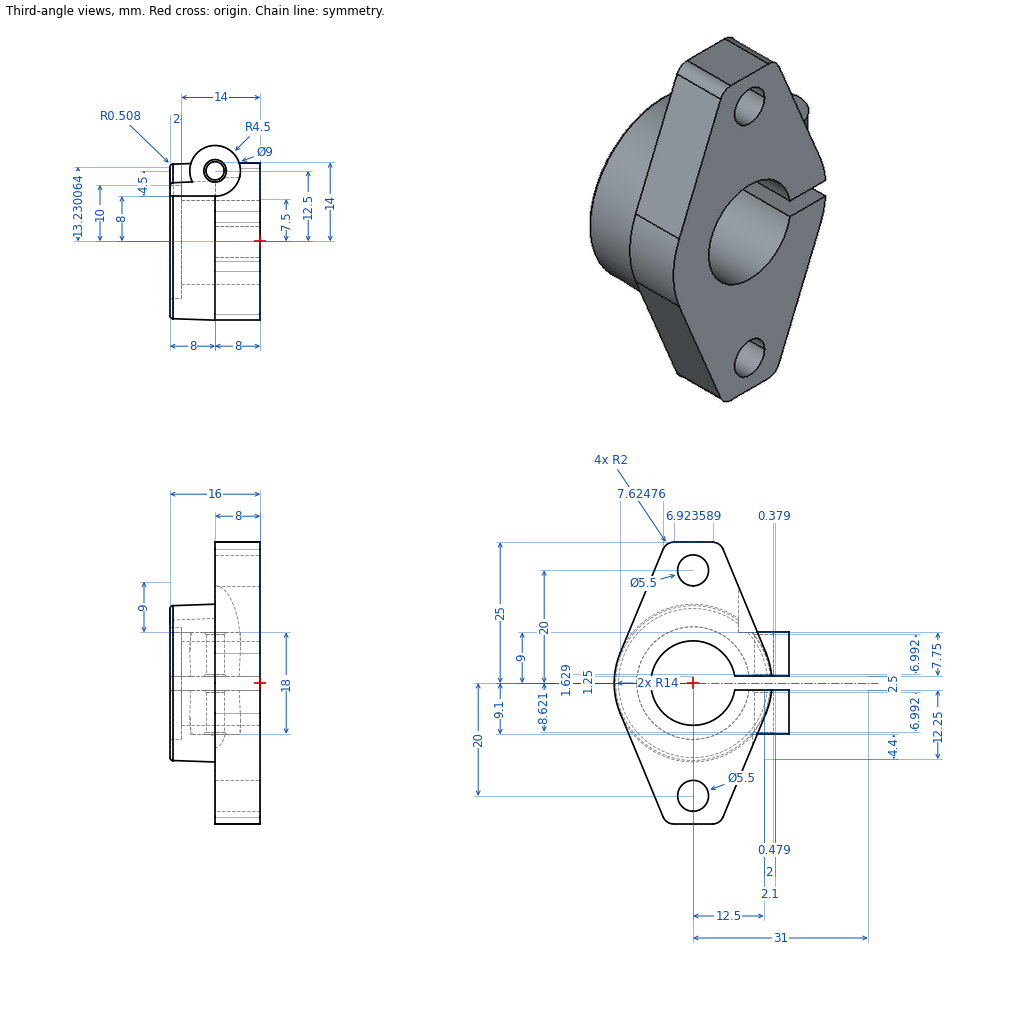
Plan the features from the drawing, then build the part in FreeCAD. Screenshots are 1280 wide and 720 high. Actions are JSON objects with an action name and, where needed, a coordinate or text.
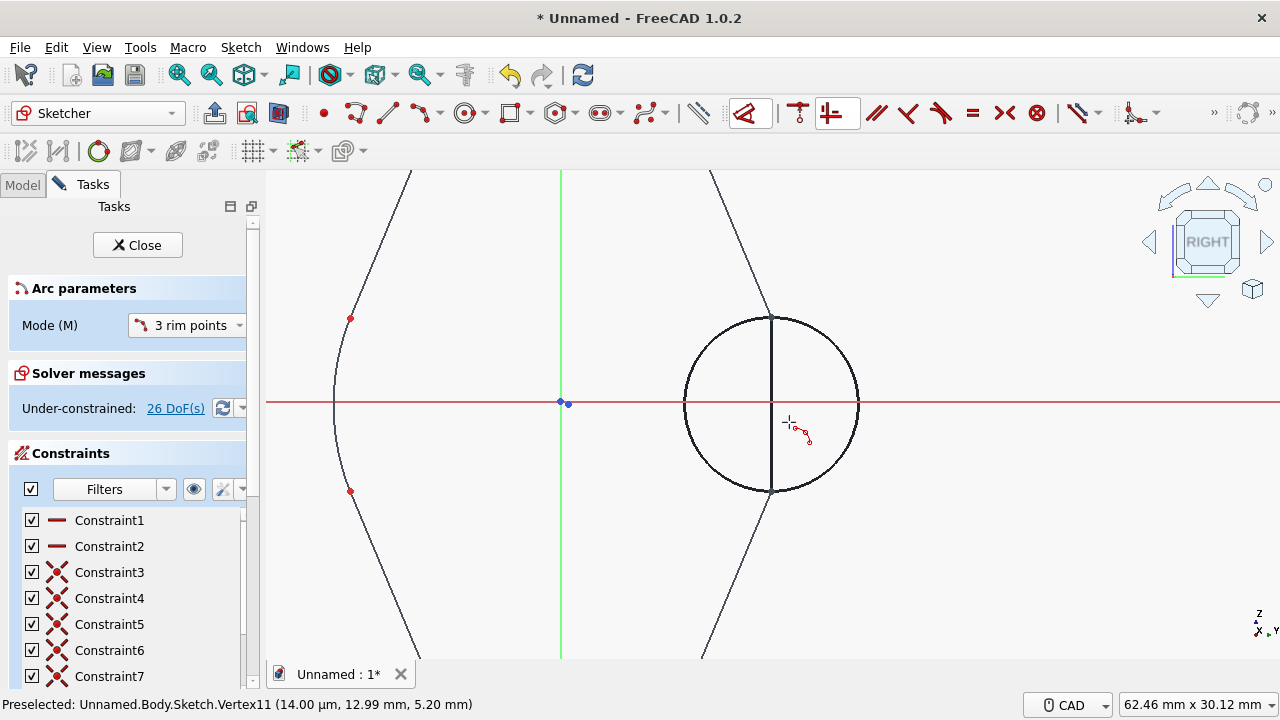
{"action": "left_click", "coordinate": [787, 420]}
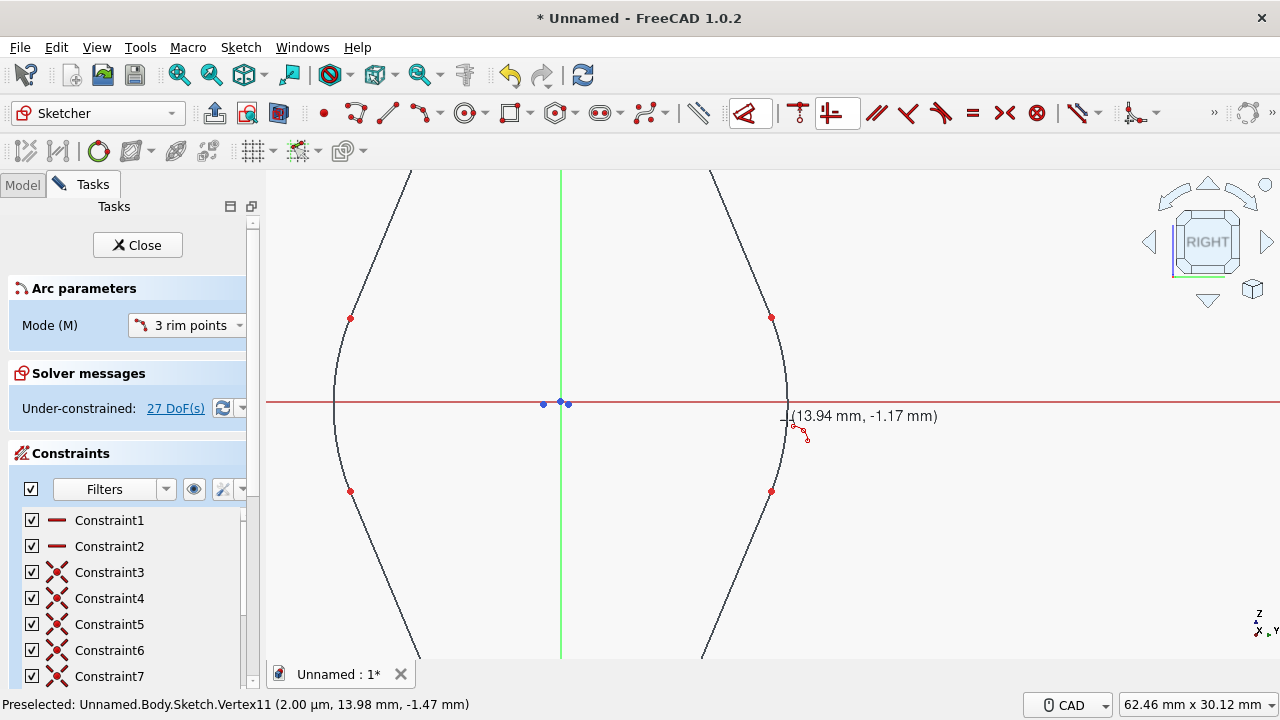
{"action": "scroll", "coordinate": [788, 422], "scroll_direction": "down", "scroll_amount": 5}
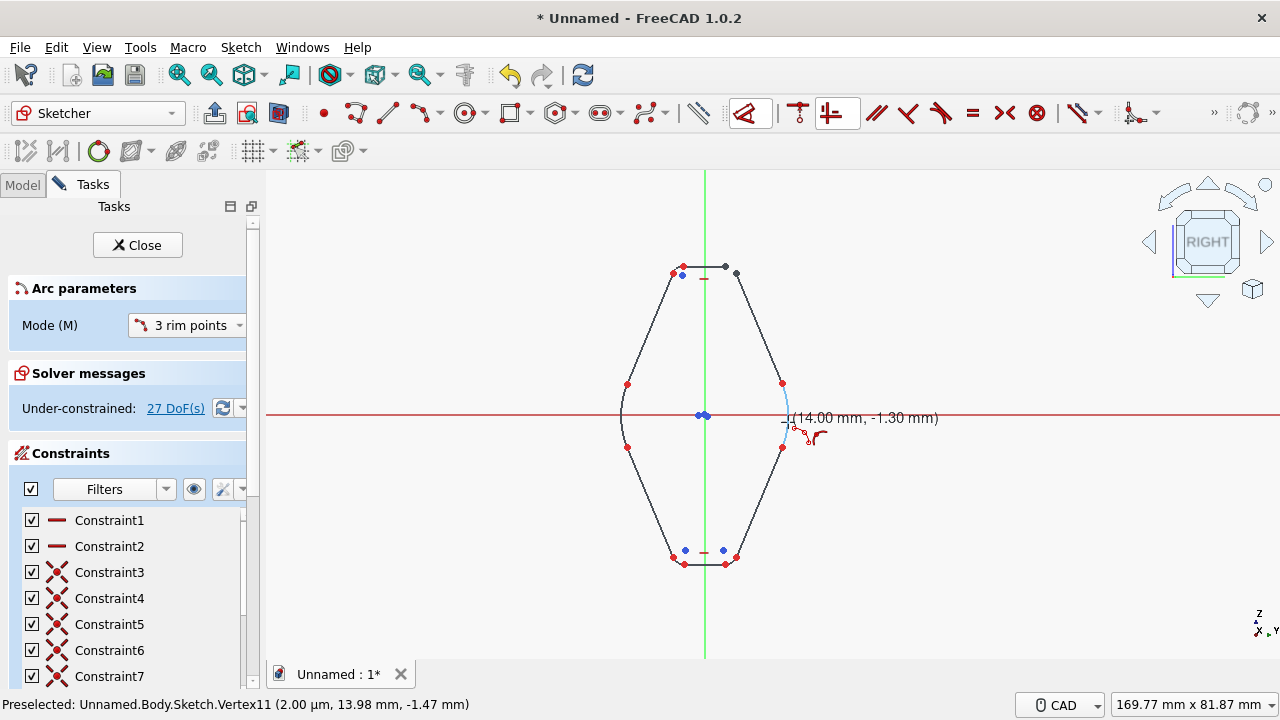
{"action": "left_click", "coordinate": [736, 274]}
{"action": "left_click", "coordinate": [725, 267]}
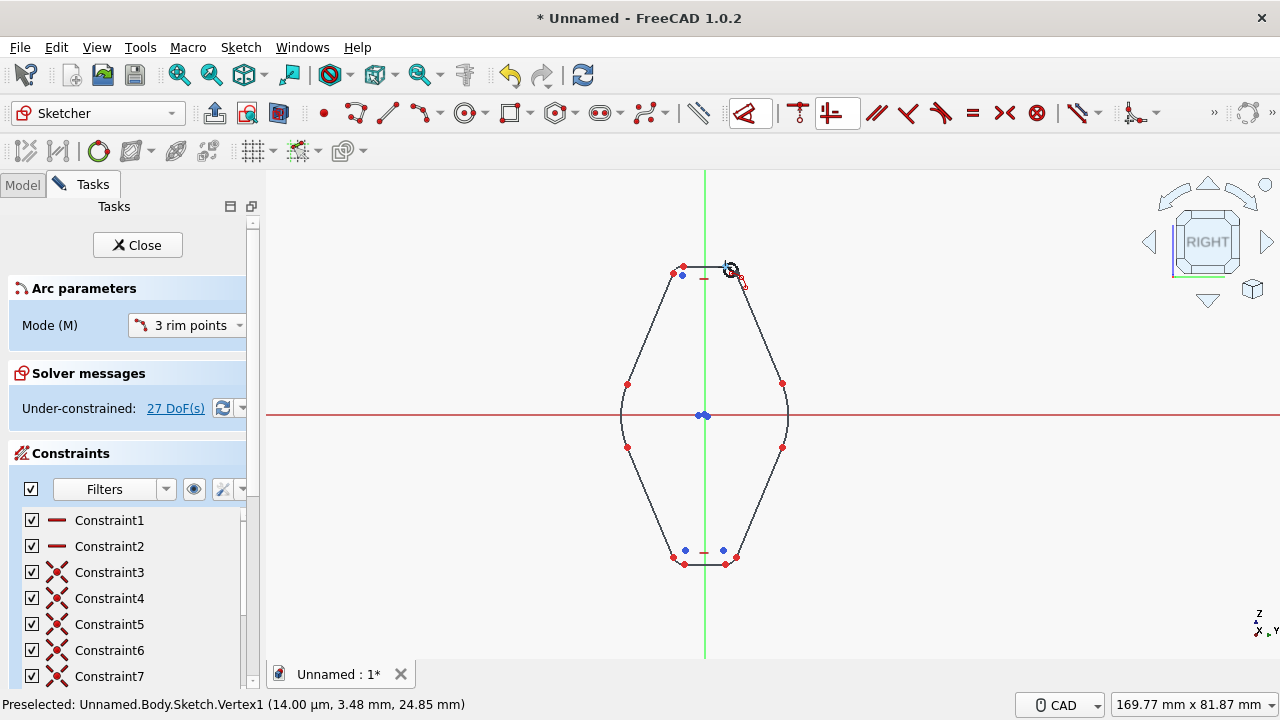
{"action": "scroll", "coordinate": [732, 268], "scroll_direction": "up", "scroll_amount": 11}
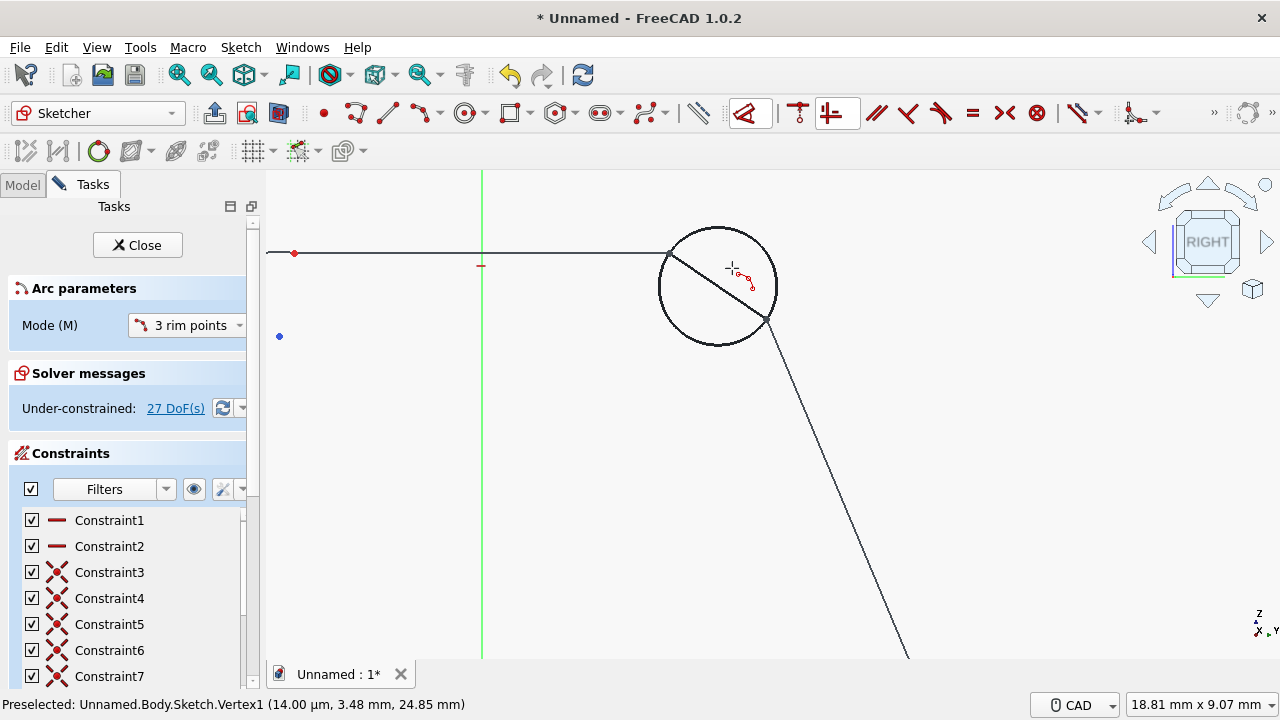
{"action": "left_click", "coordinate": [728, 263]}
{"action": "key", "text": "Escape"}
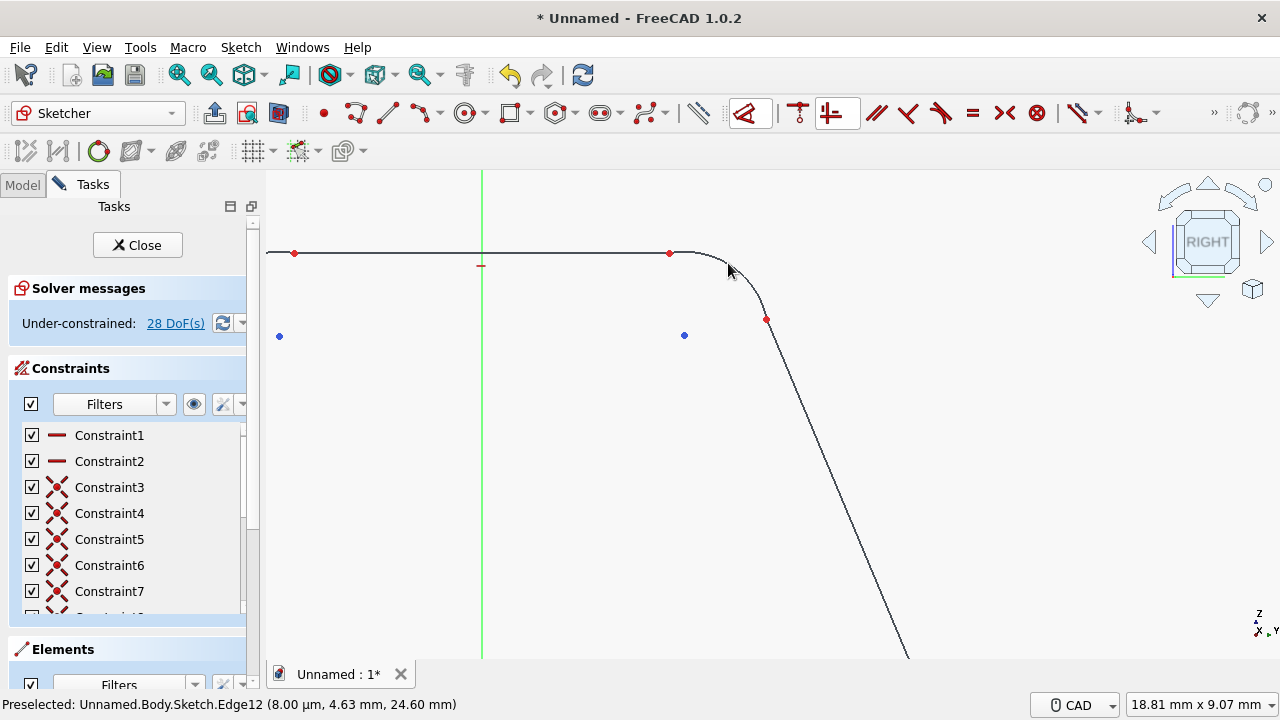
{"action": "scroll", "coordinate": [732, 268], "scroll_direction": "down", "scroll_amount": 11}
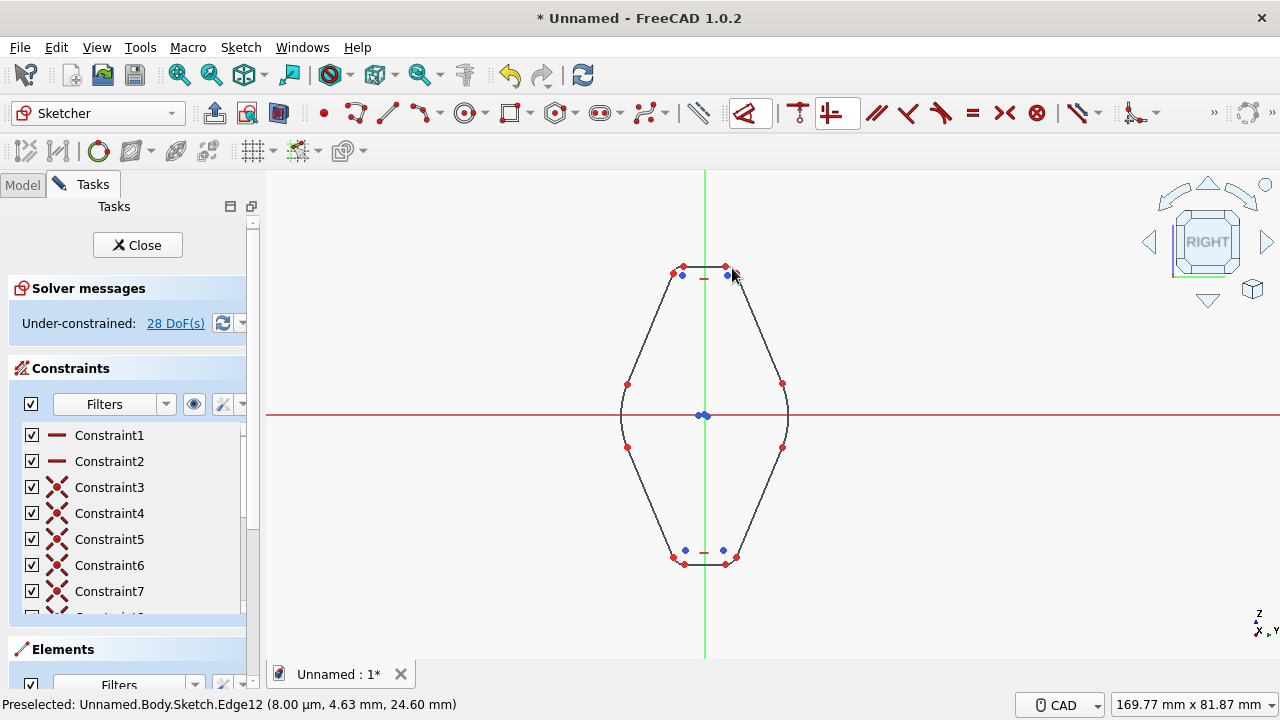
{"action": "scroll", "coordinate": [713, 267], "scroll_direction": "up", "scroll_amount": 3}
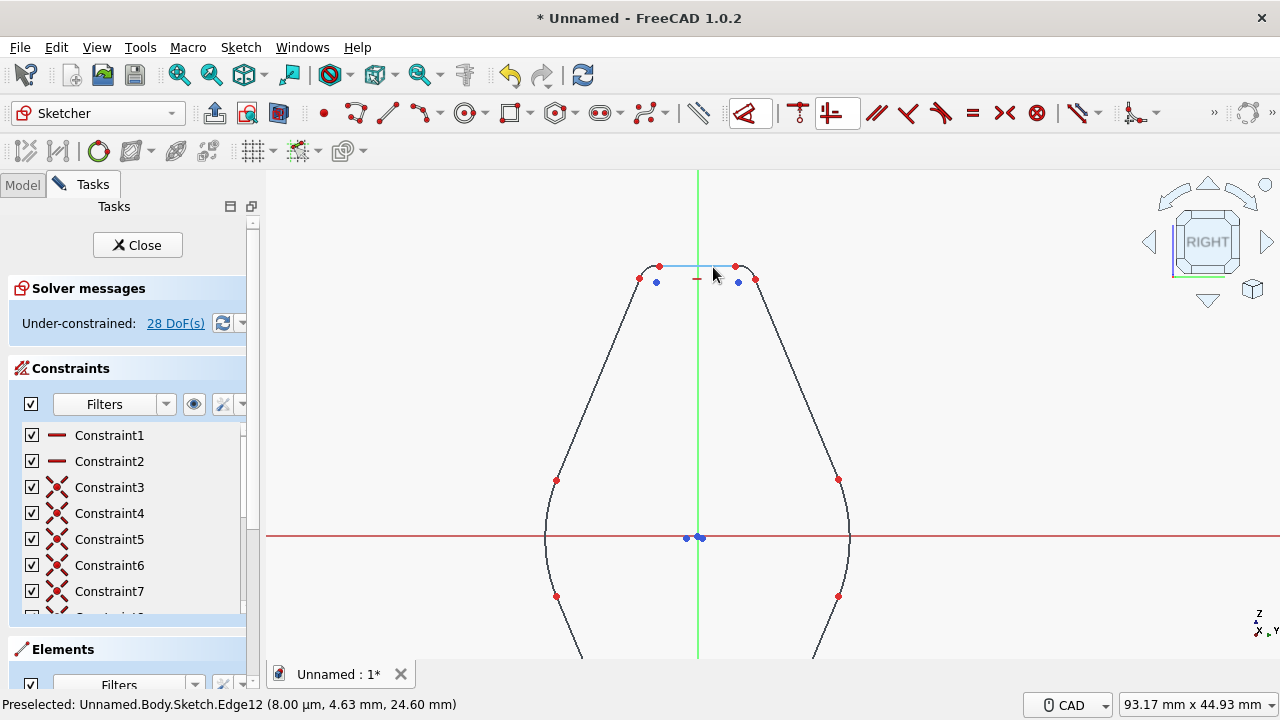
{"action": "left_click", "coordinate": [713, 266]}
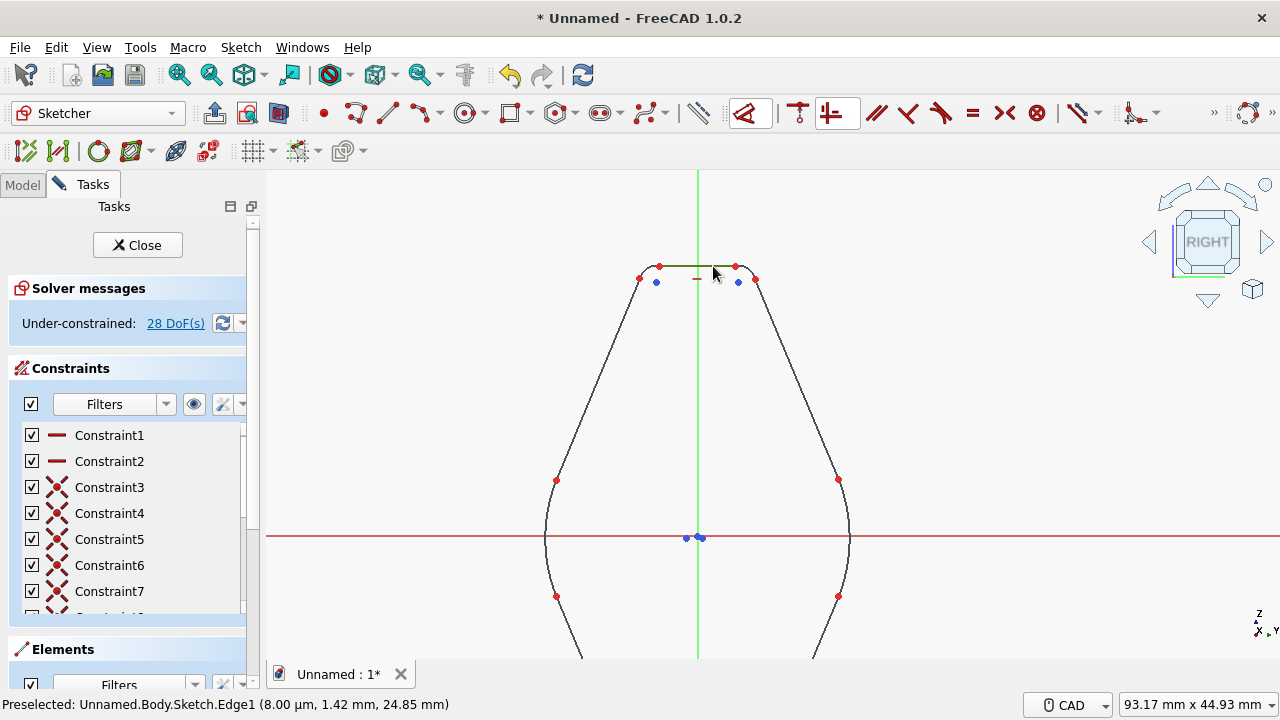
{"action": "left_click", "coordinate": [647, 268]}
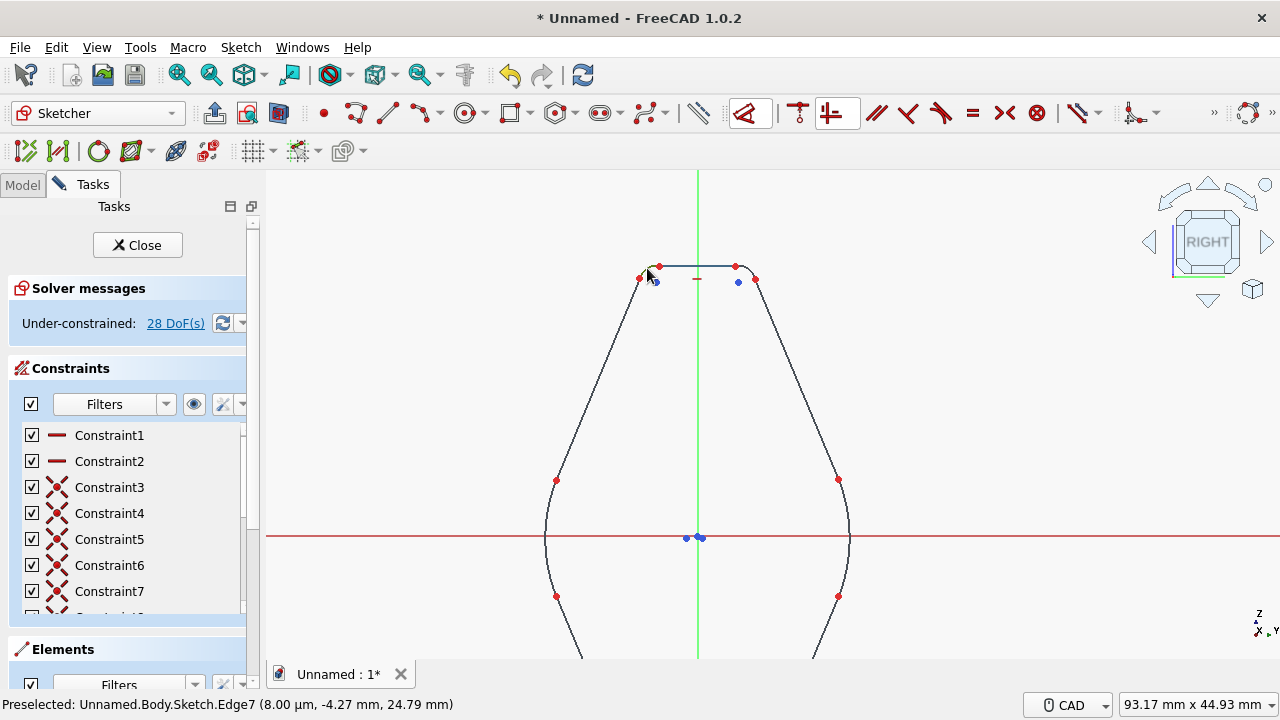
{"action": "left_click", "coordinate": [942, 114]}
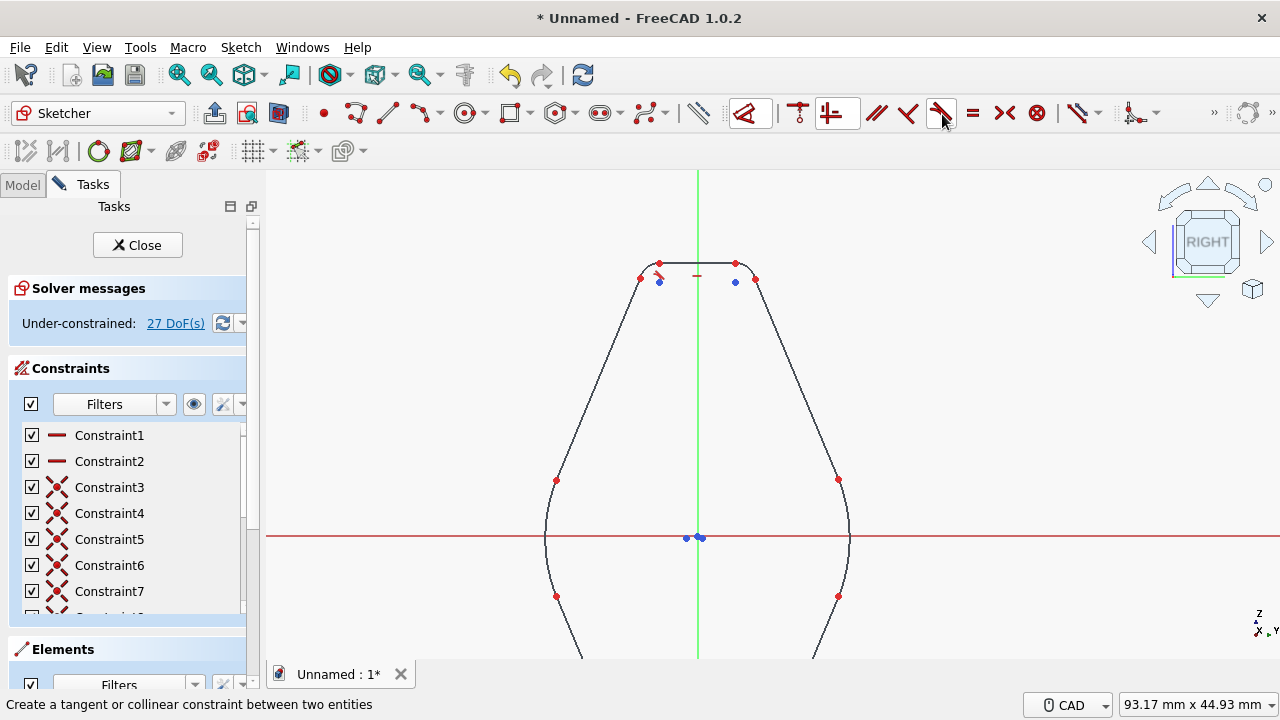
{"action": "left_click", "coordinate": [713, 263]}